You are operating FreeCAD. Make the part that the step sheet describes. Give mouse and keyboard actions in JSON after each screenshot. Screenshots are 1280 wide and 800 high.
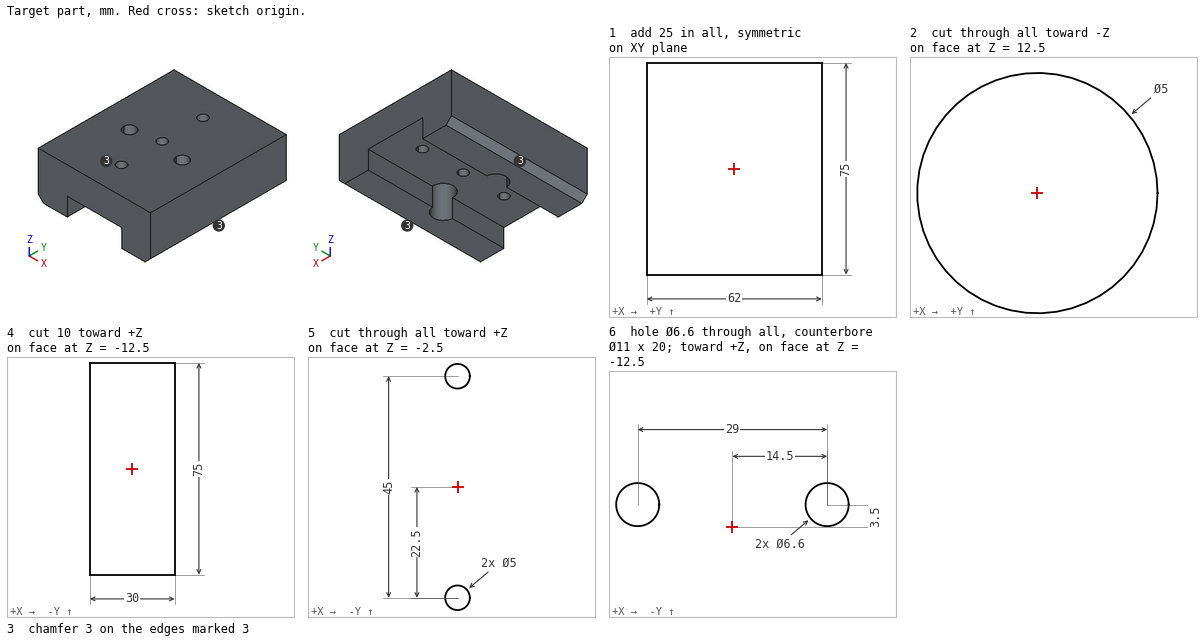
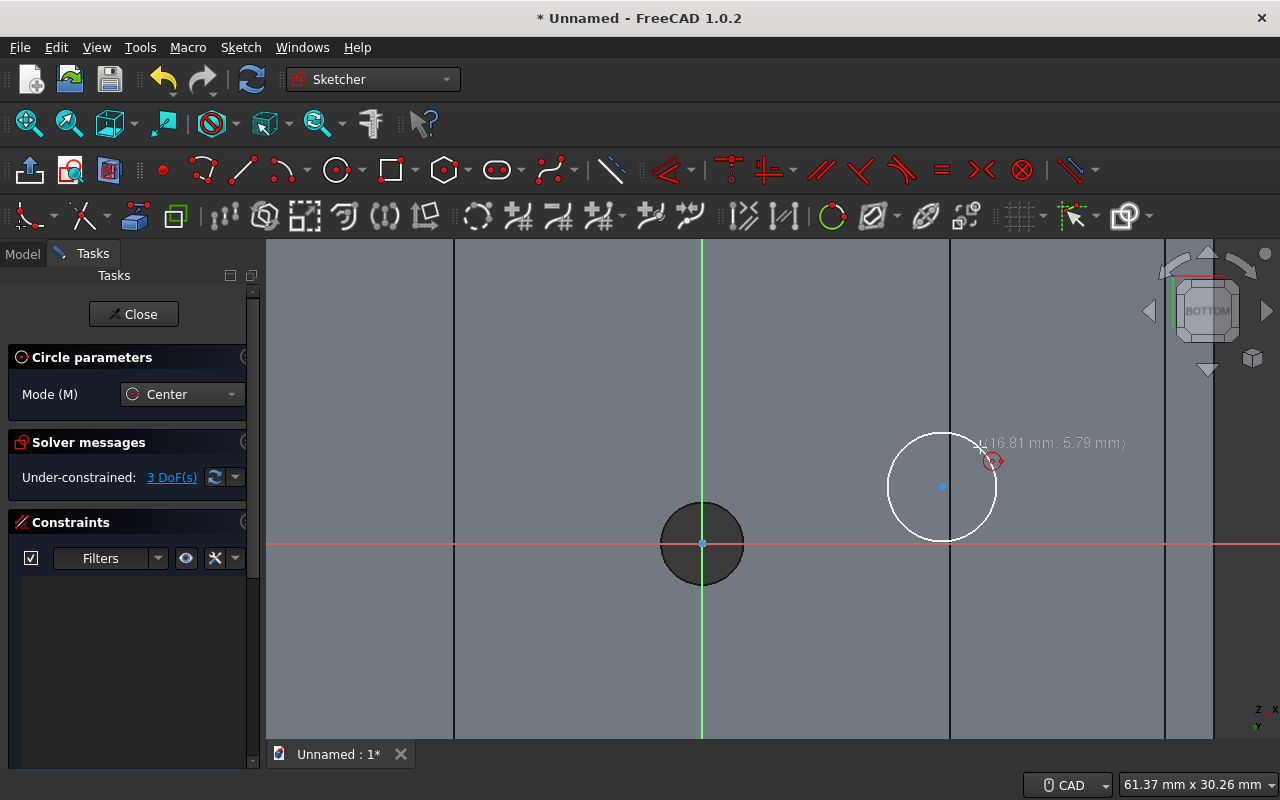
{"action": "left_click", "coordinate": [463, 486]}
{"action": "left_click", "coordinate": [501, 447]}
{"action": "key", "text": "Escape"}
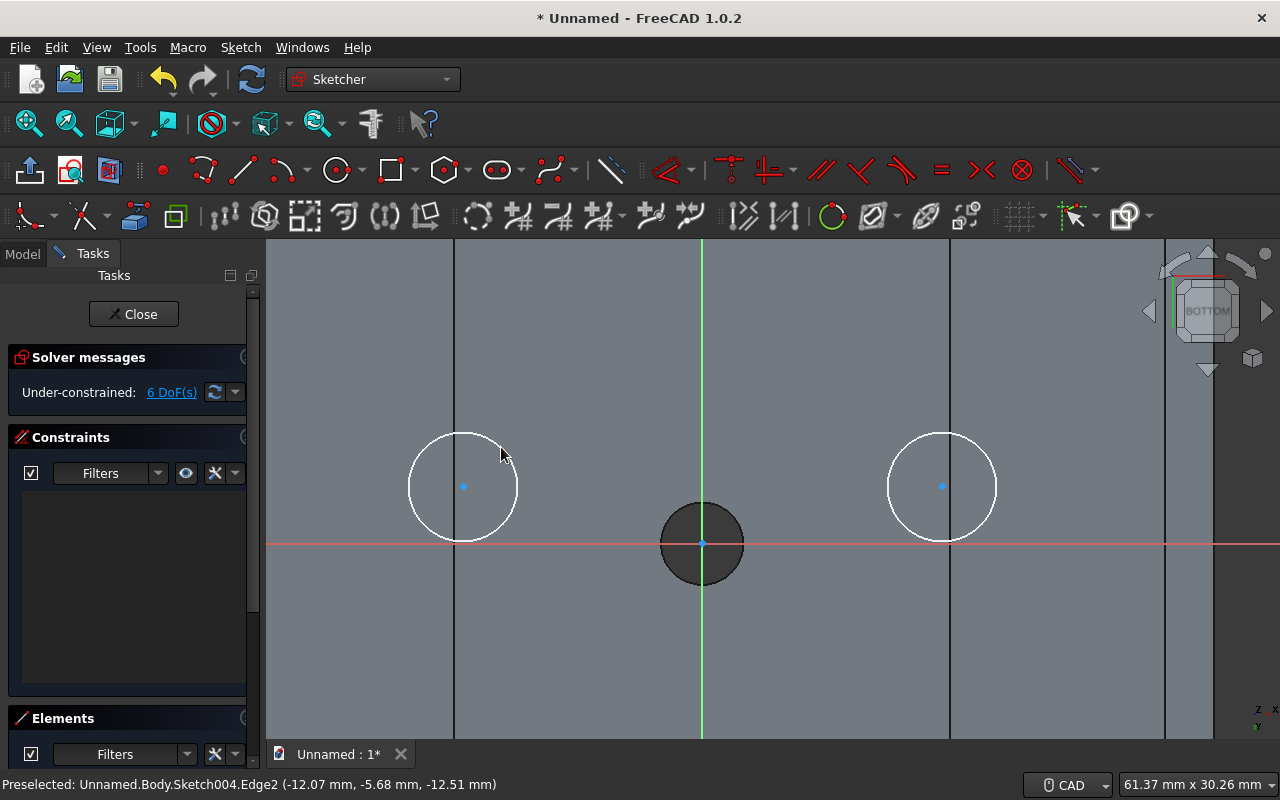
{"action": "left_click", "coordinate": [980, 448]}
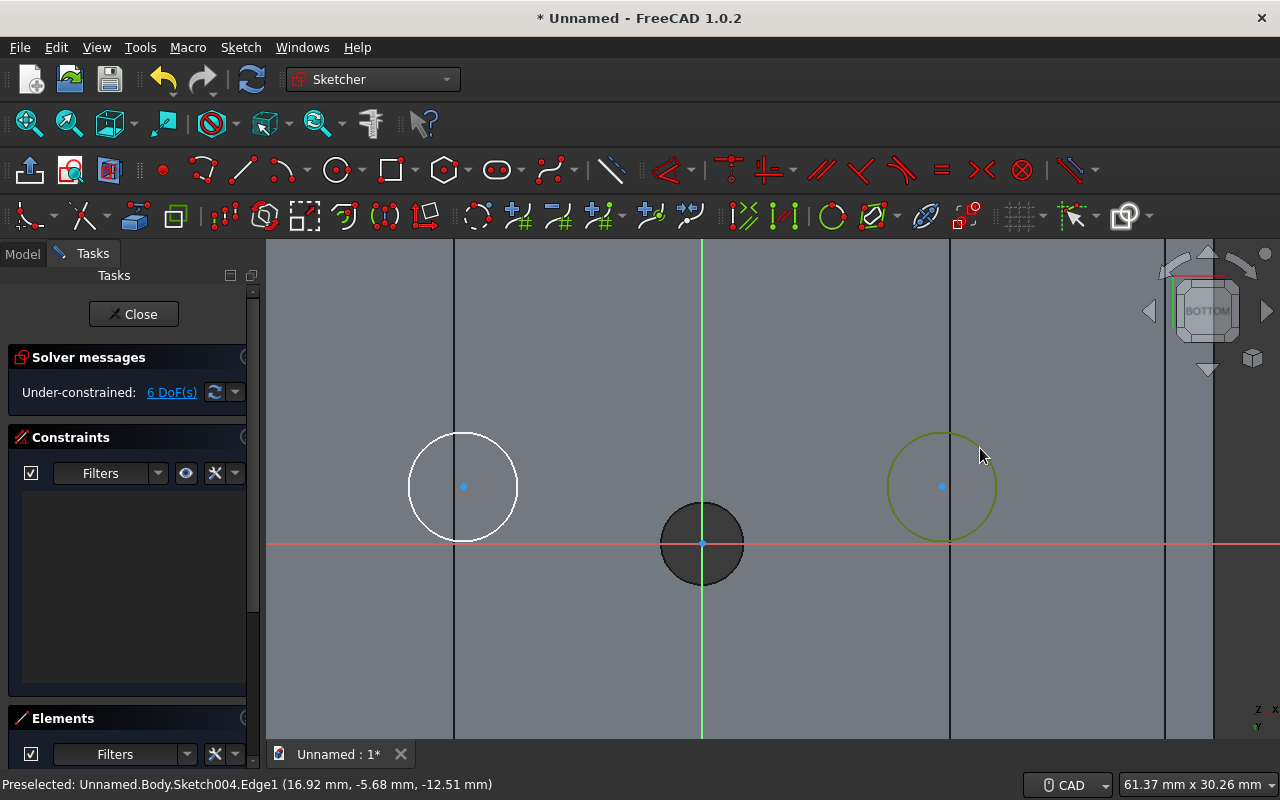
{"action": "left_click", "coordinate": [501, 448]}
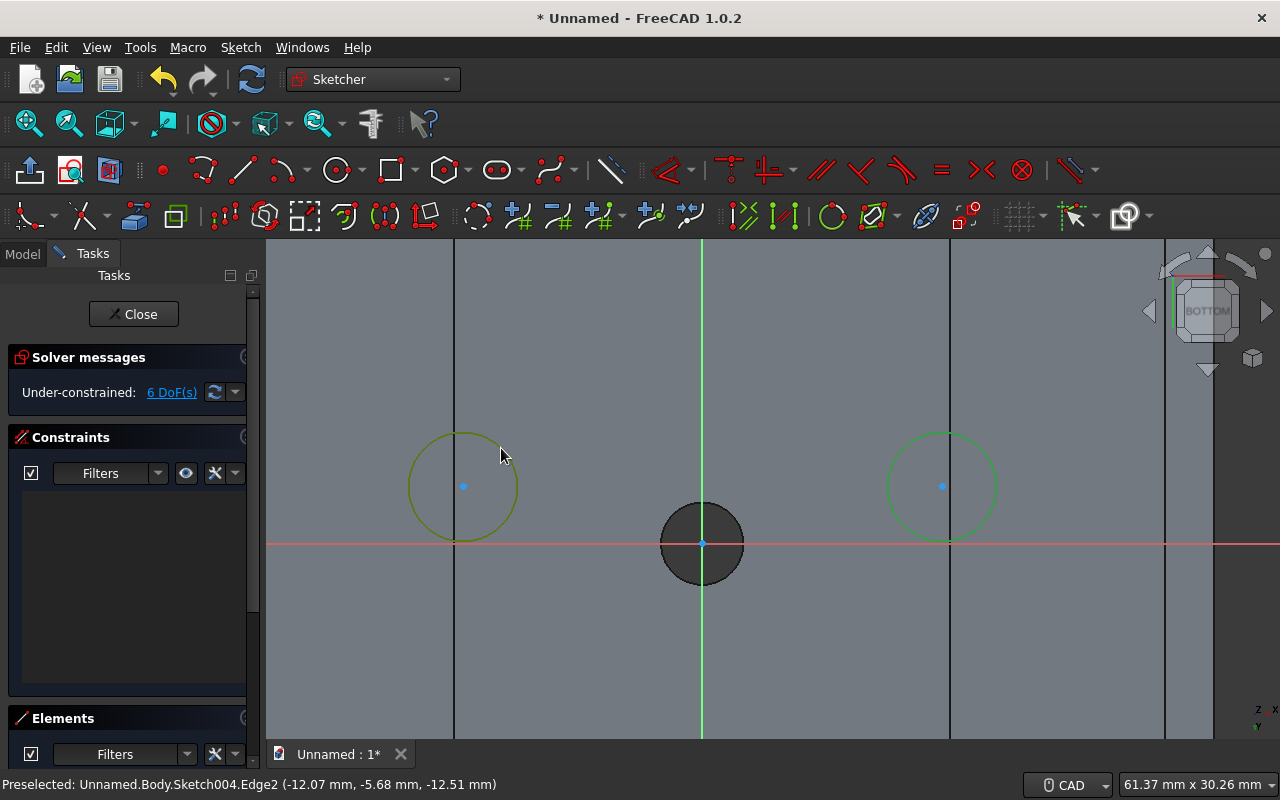
{"action": "left_click", "coordinate": [942, 170]}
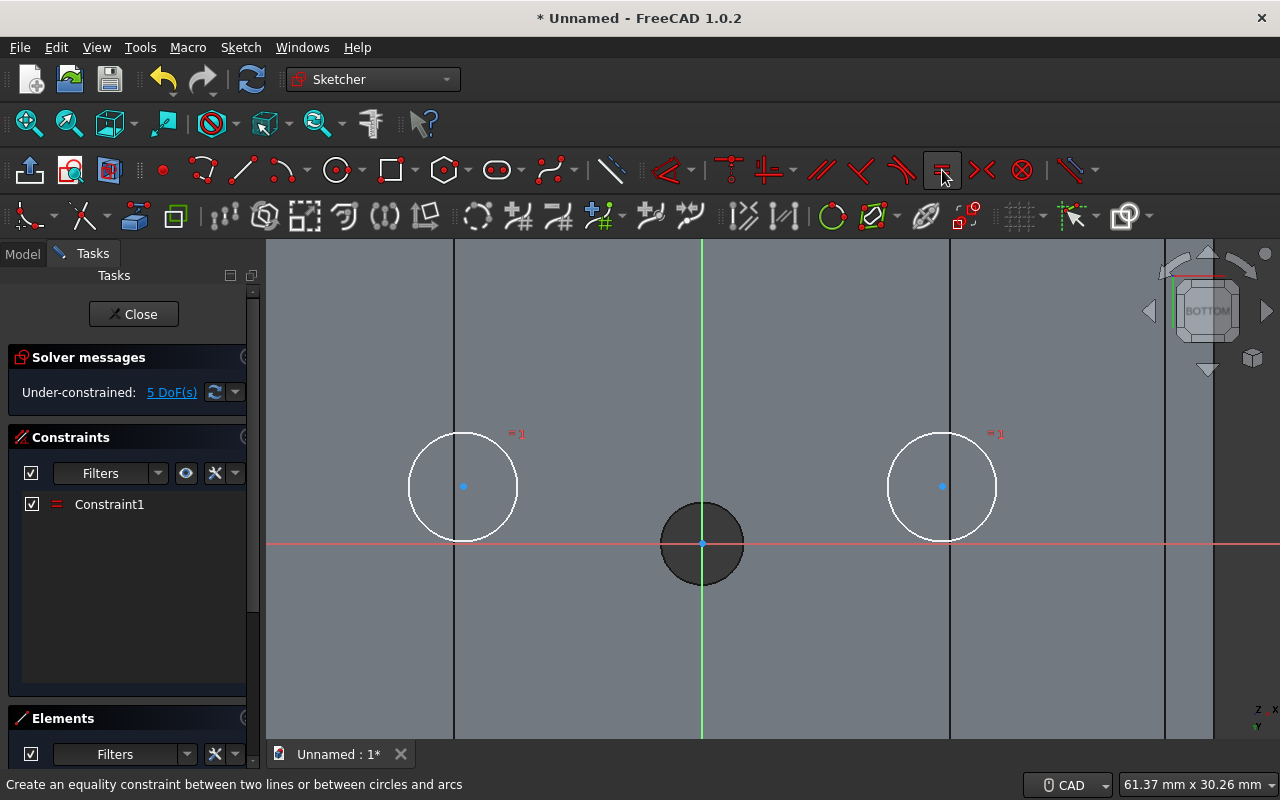
{"action": "left_click", "coordinate": [942, 487]}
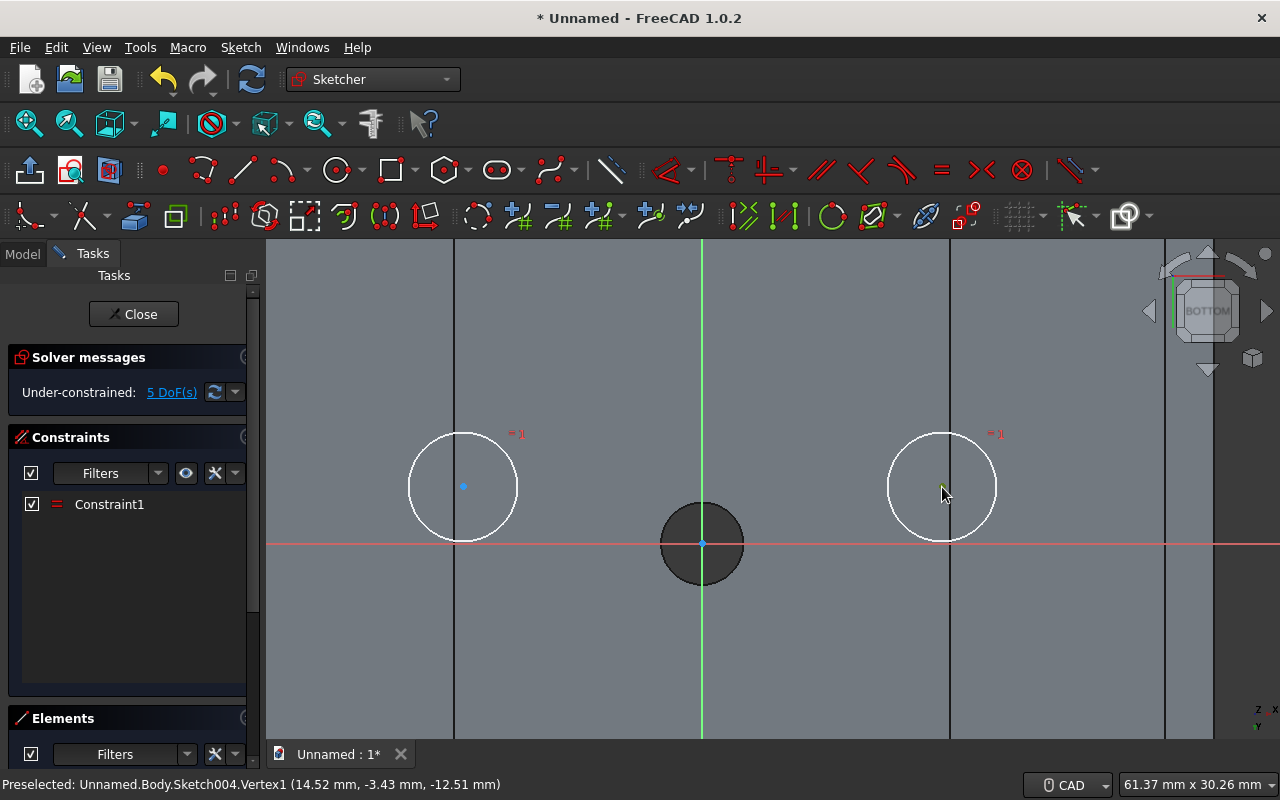
{"action": "left_click", "coordinate": [463, 487]}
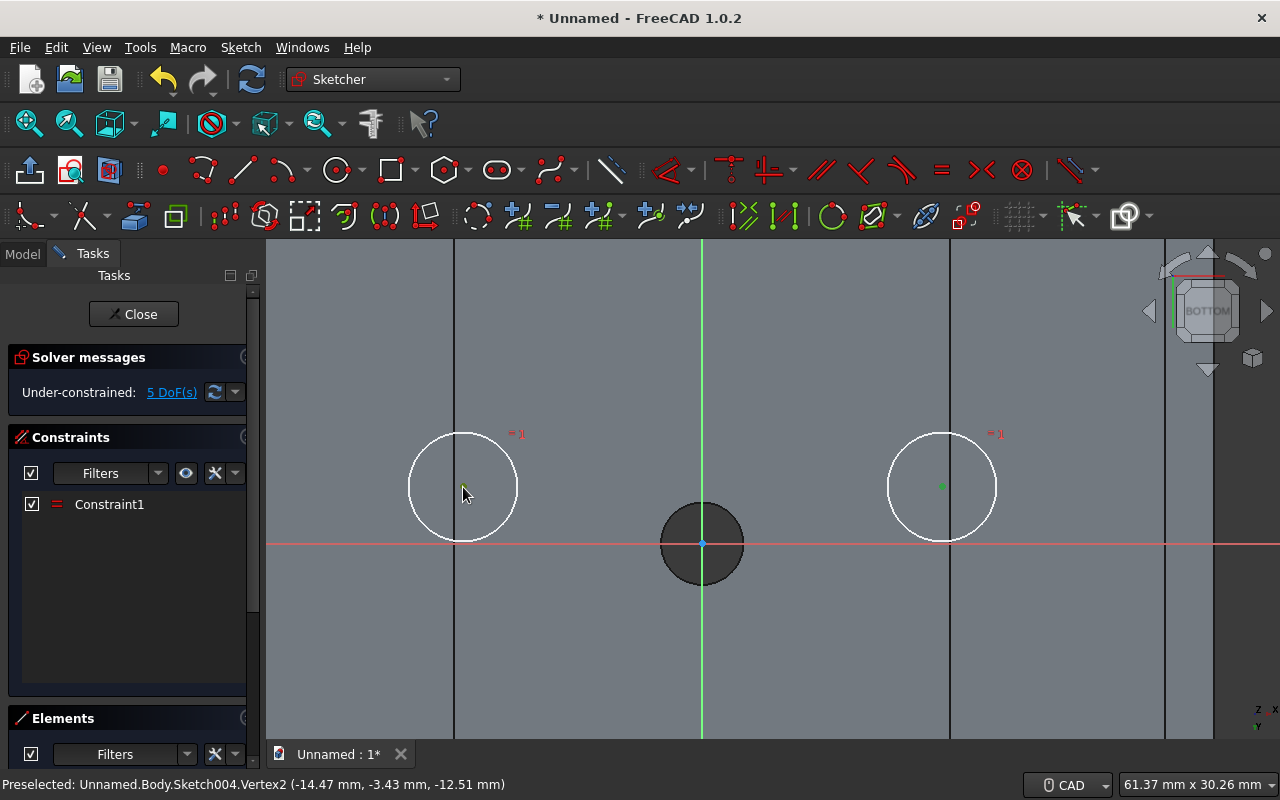
{"action": "key", "text": "h"}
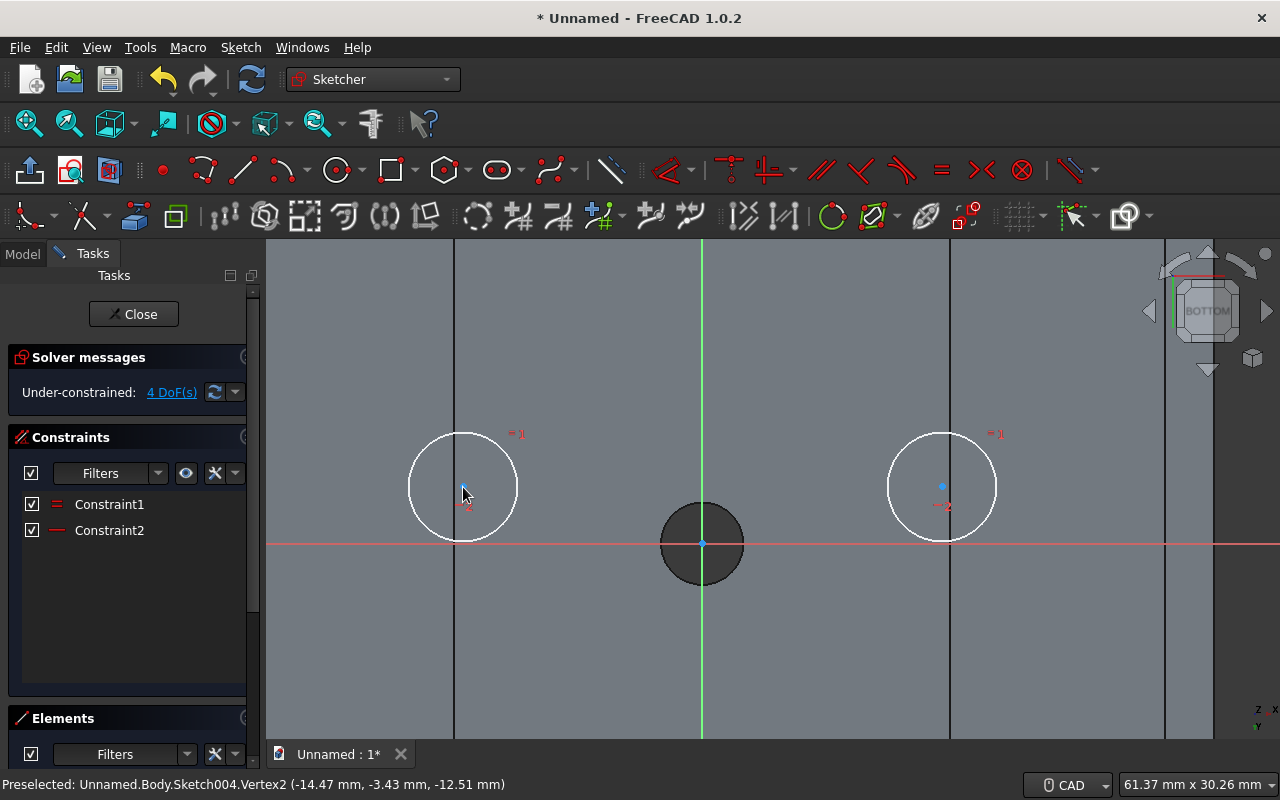
{"action": "key", "text": "d"}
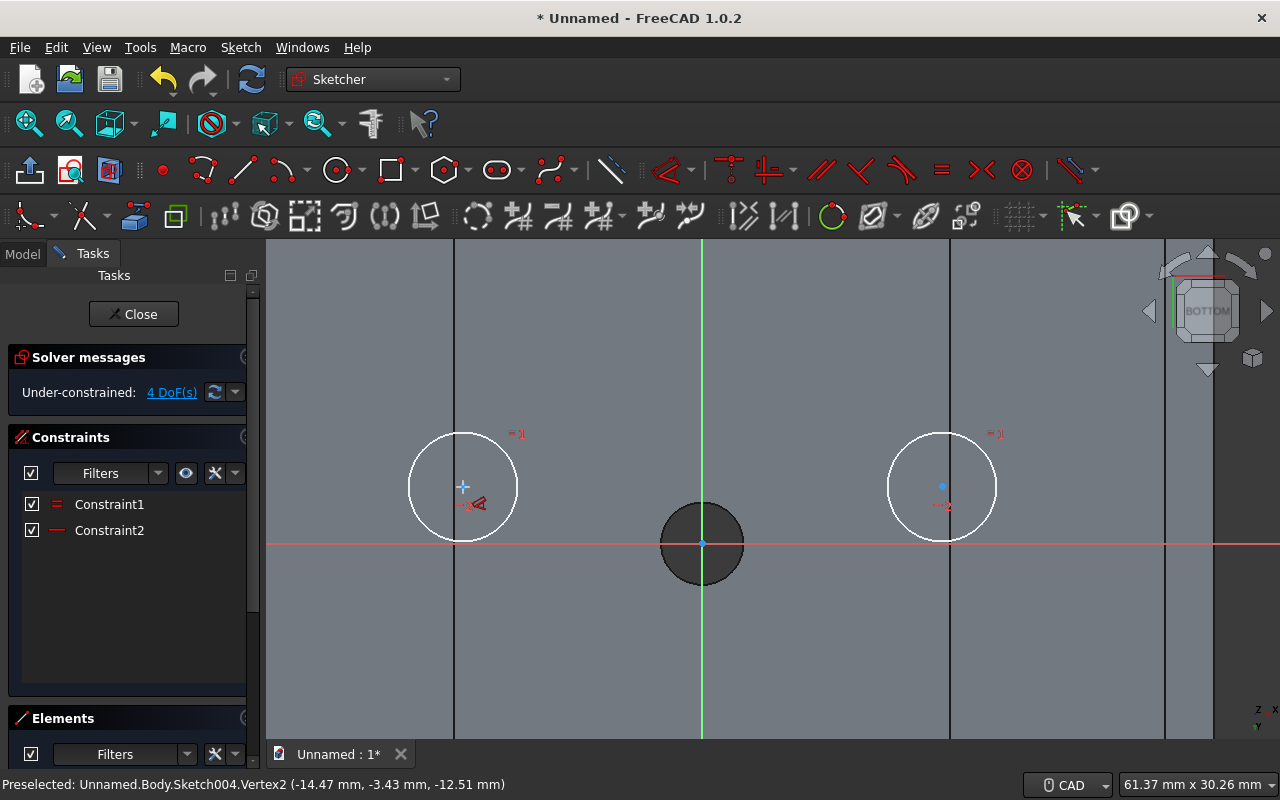
{"action": "left_click", "coordinate": [980, 448]}
{"action": "left_click", "coordinate": [1002, 425]}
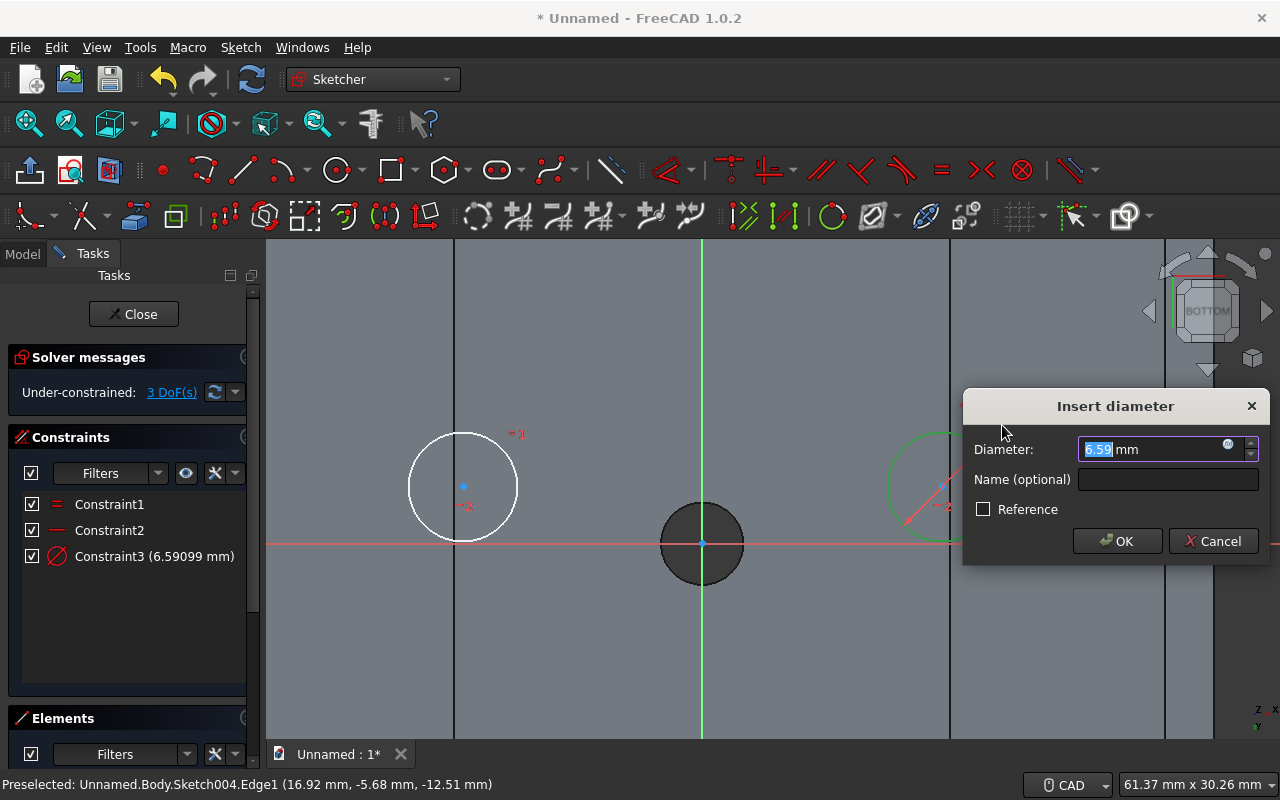
{"action": "type", "text": "6.6"}
{"action": "key", "text": "Return"}